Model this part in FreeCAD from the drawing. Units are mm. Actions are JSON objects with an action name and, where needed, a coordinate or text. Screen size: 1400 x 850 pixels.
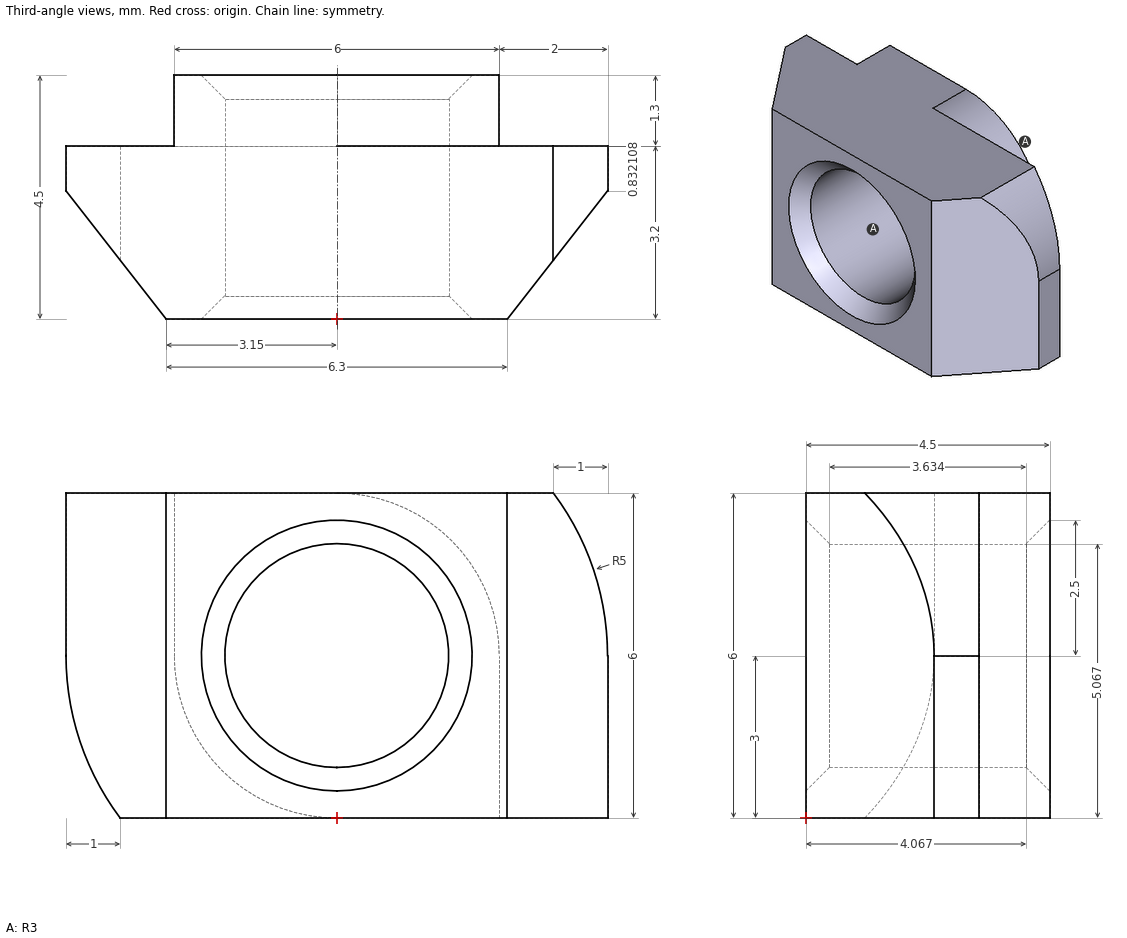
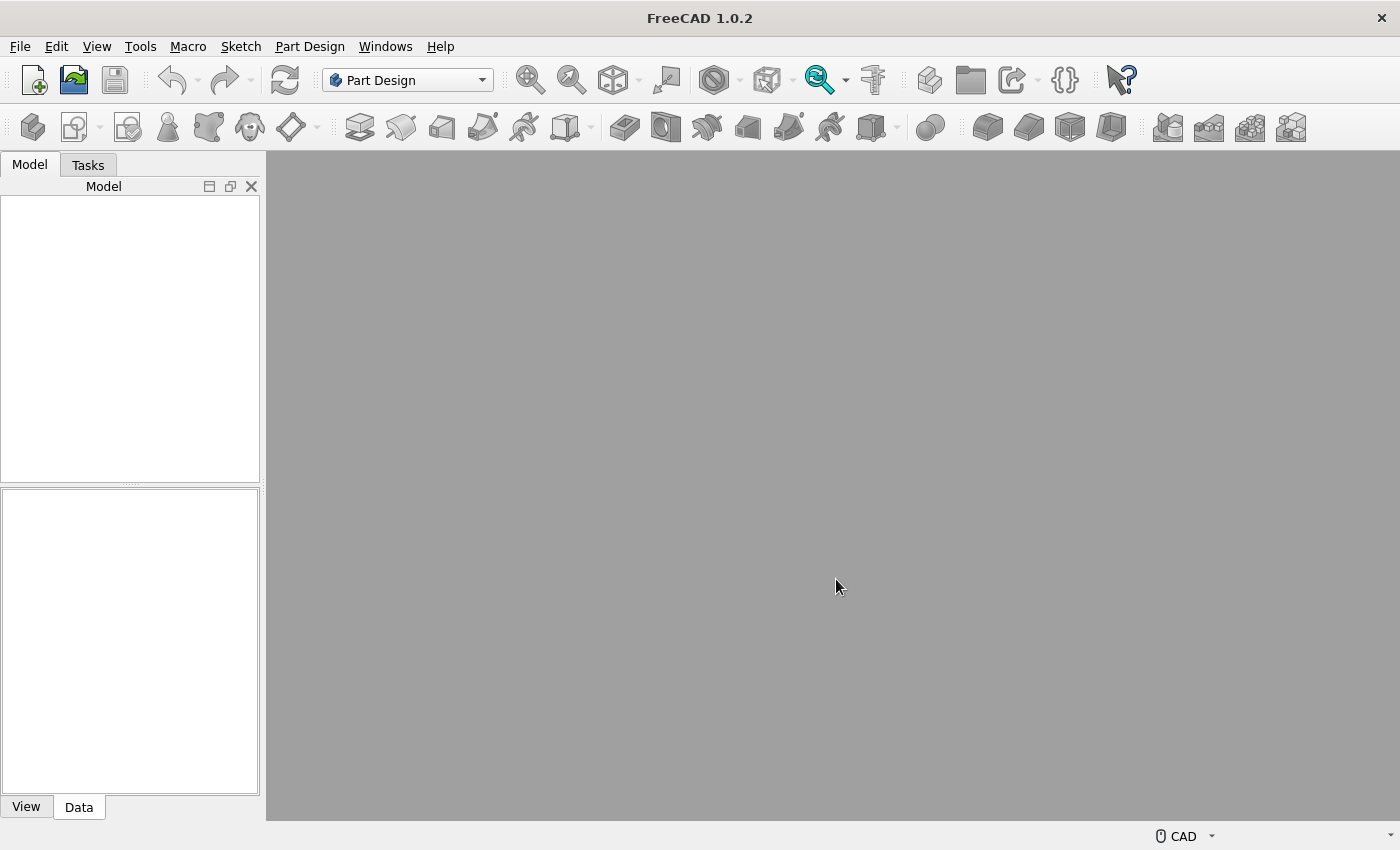
{"action": "left_click", "coordinate": [33, 80]}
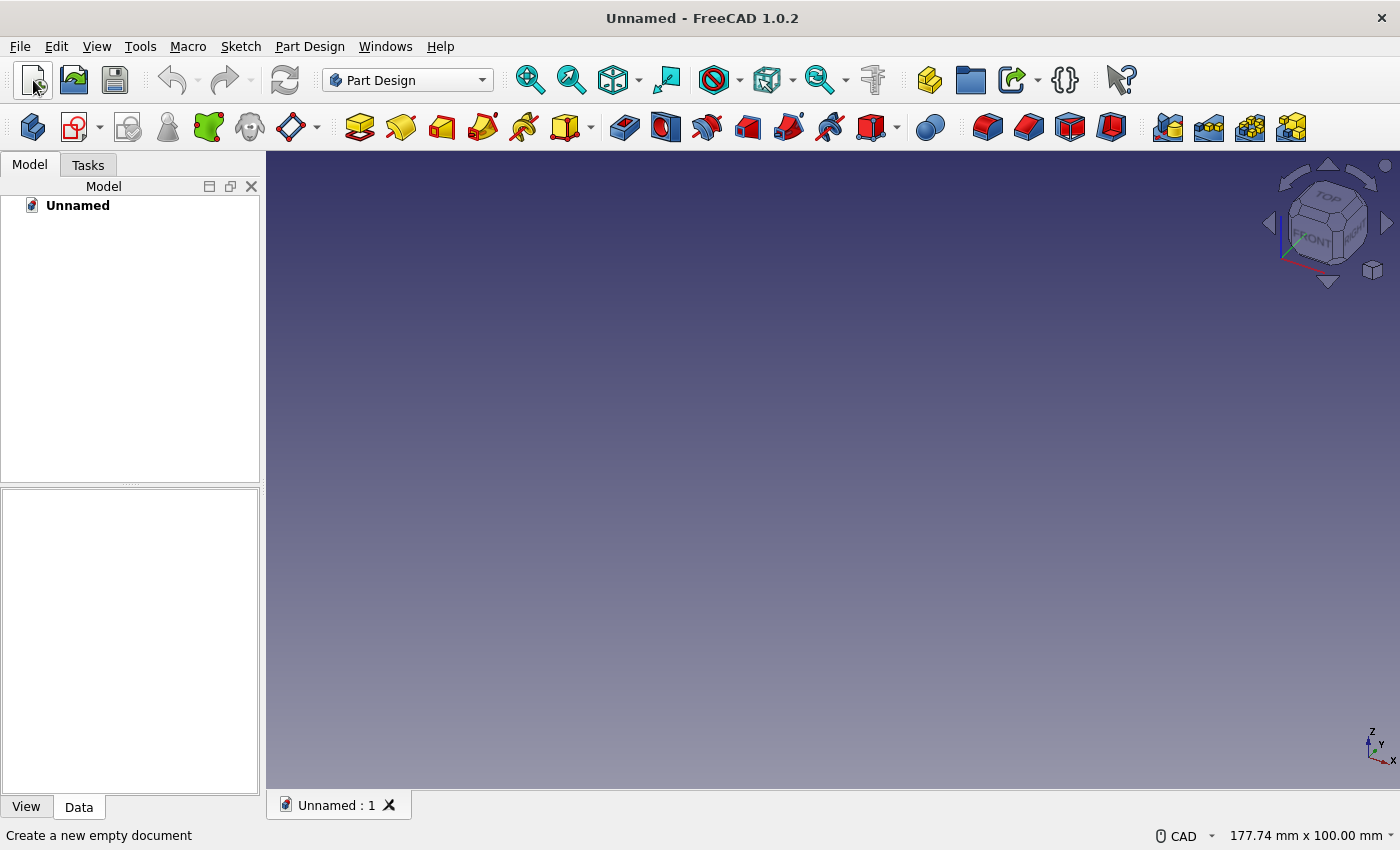
{"action": "left_click", "coordinate": [74, 128]}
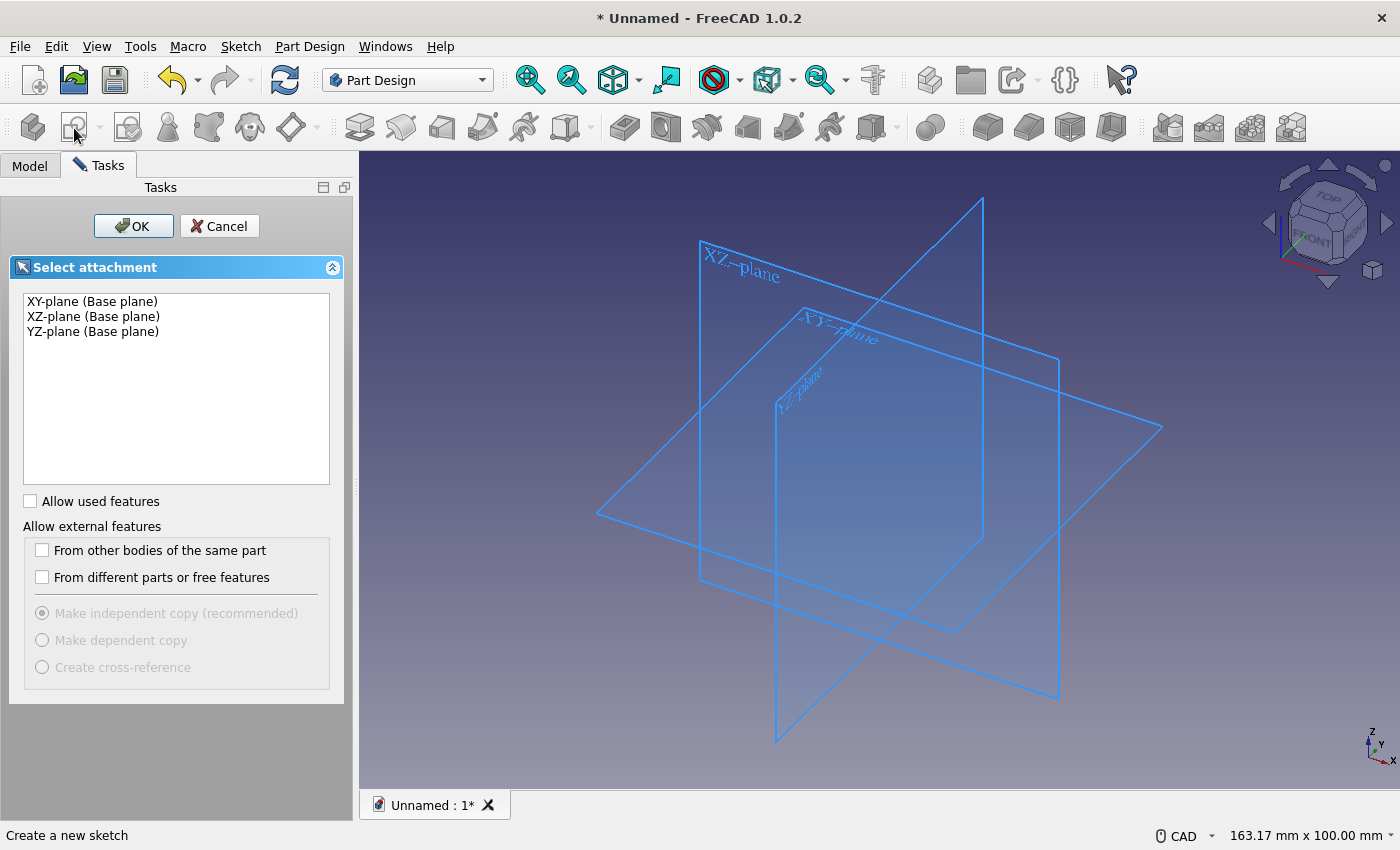
{"action": "left_click", "coordinate": [84, 302]}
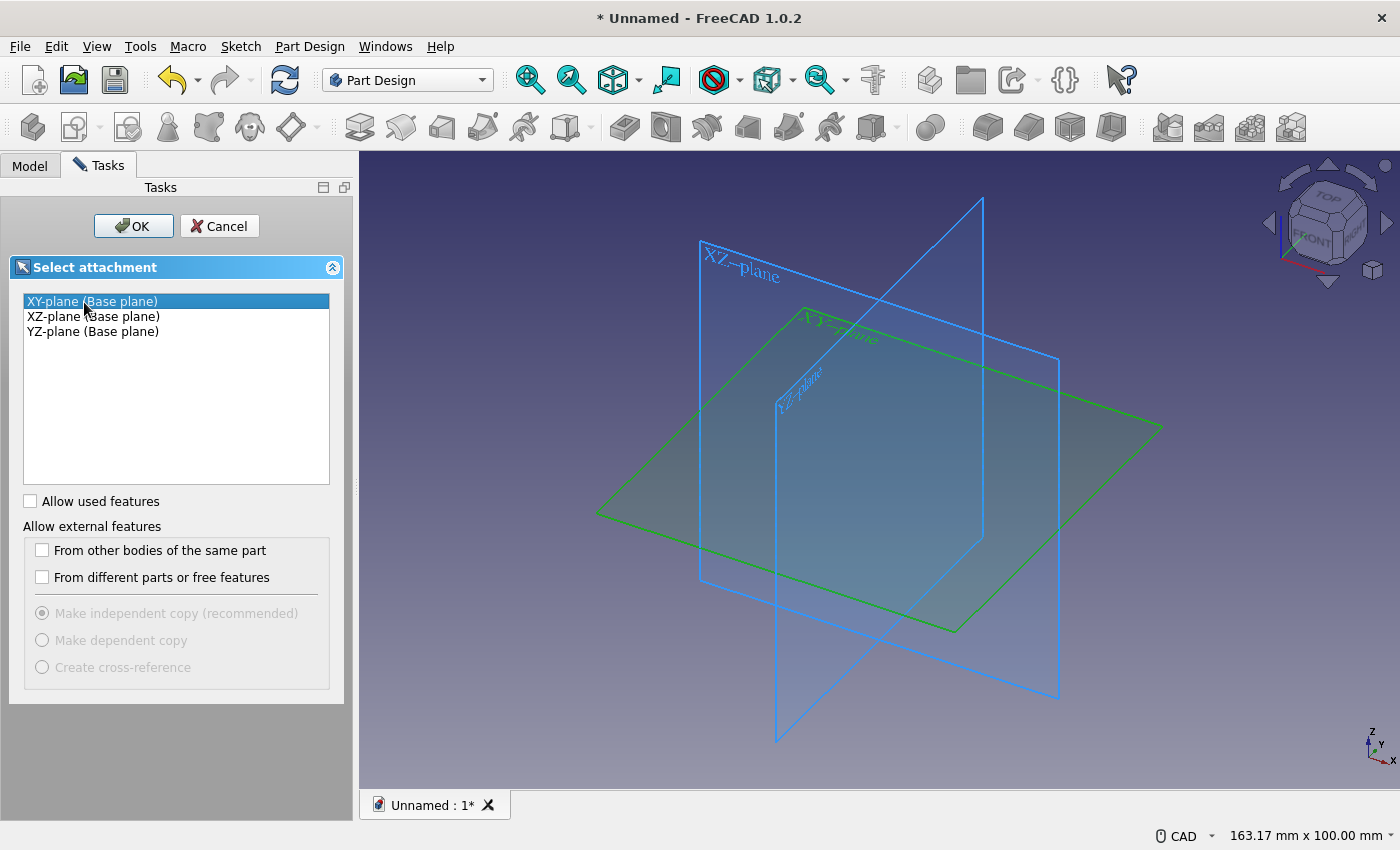
{"action": "left_click", "coordinate": [134, 226]}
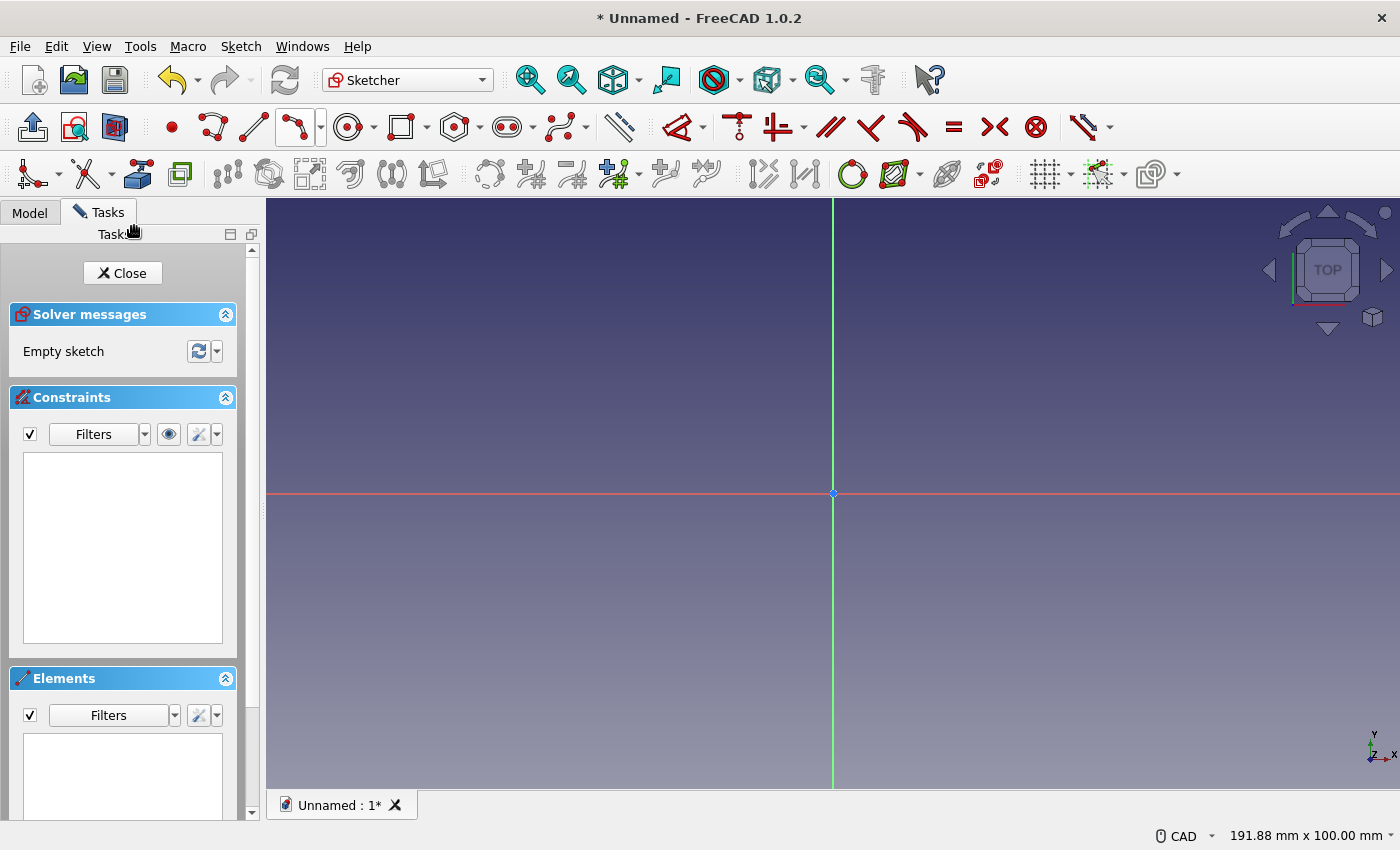
{"action": "scroll", "coordinate": [840, 479], "scroll_direction": "up", "scroll_amount": 12}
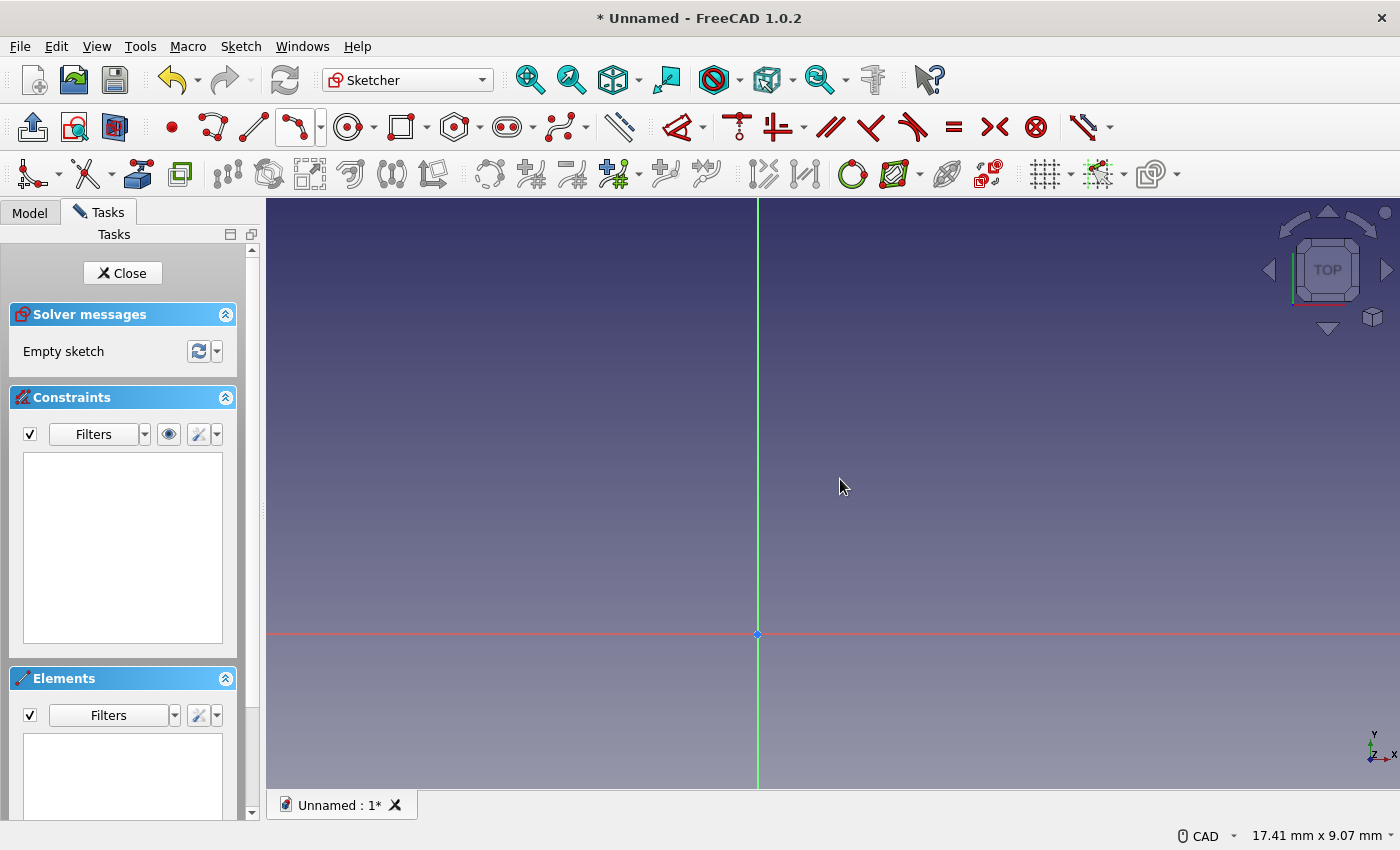
{"action": "left_click", "coordinate": [213, 128]}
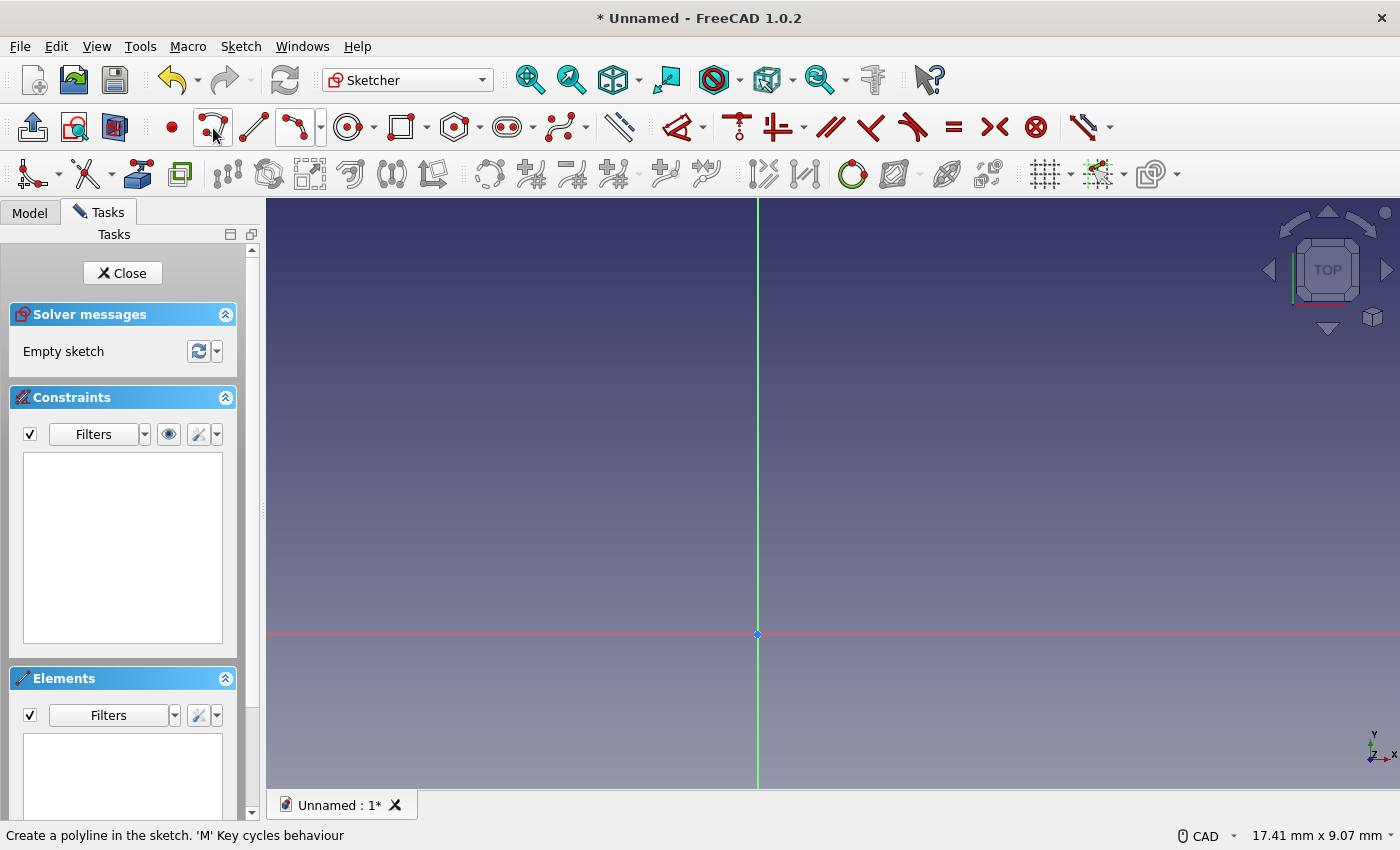
{"action": "left_click", "coordinate": [553, 634]}
{"action": "left_click", "coordinate": [963, 625]}
{"action": "left_click", "coordinate": [1083, 480]}
{"action": "left_click", "coordinate": [1083, 426]}
{"action": "left_click", "coordinate": [953, 426]}
{"action": "left_click", "coordinate": [953, 341]}
{"action": "left_click", "coordinate": [562, 341]}
{"action": "left_click", "coordinate": [562, 426]}
{"action": "left_click", "coordinate": [432, 426]}
{"action": "left_click", "coordinate": [432, 480]}
{"action": "left_click", "coordinate": [553, 634]}
{"action": "key", "text": "Escape"}
{"action": "key", "text": "Escape"}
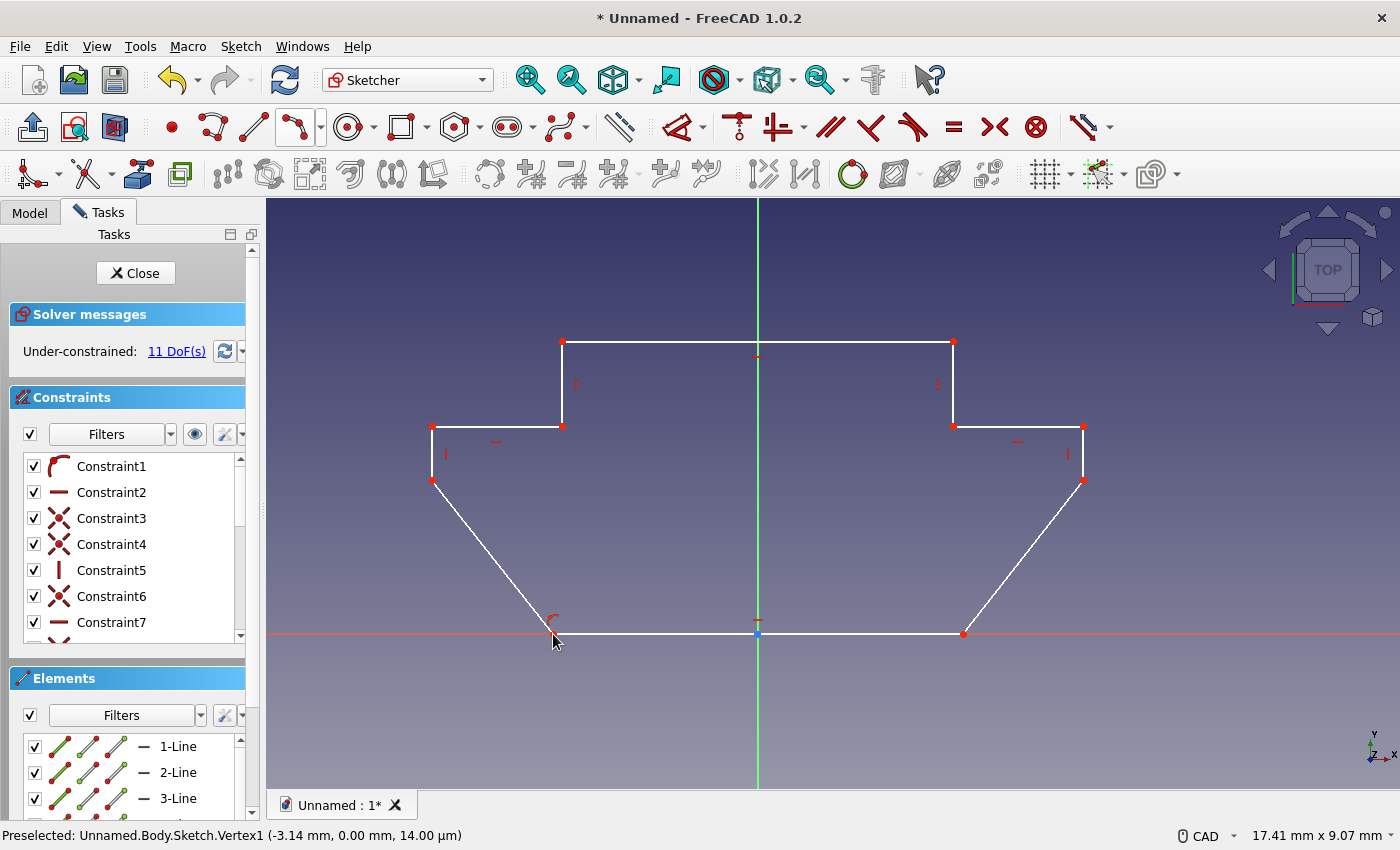
{"action": "left_click", "coordinate": [953, 427]}